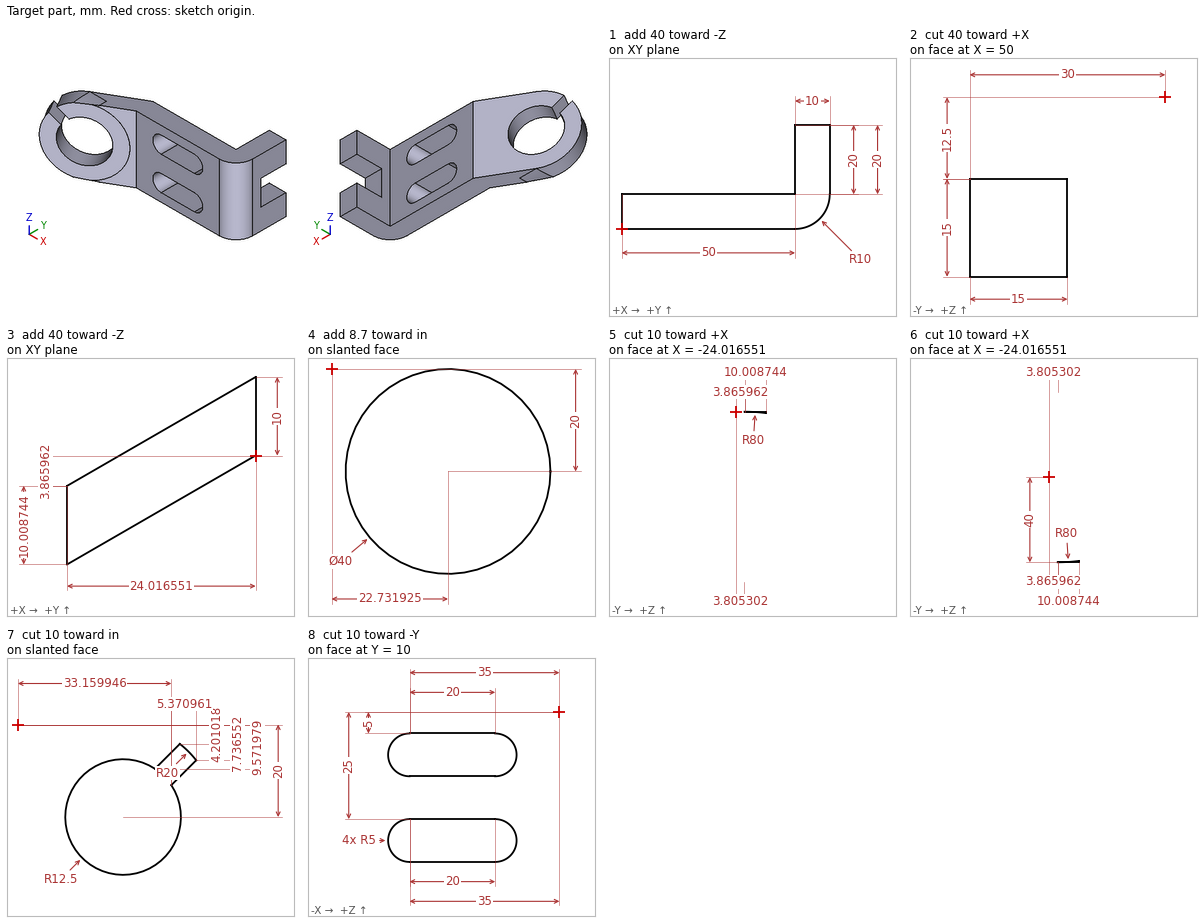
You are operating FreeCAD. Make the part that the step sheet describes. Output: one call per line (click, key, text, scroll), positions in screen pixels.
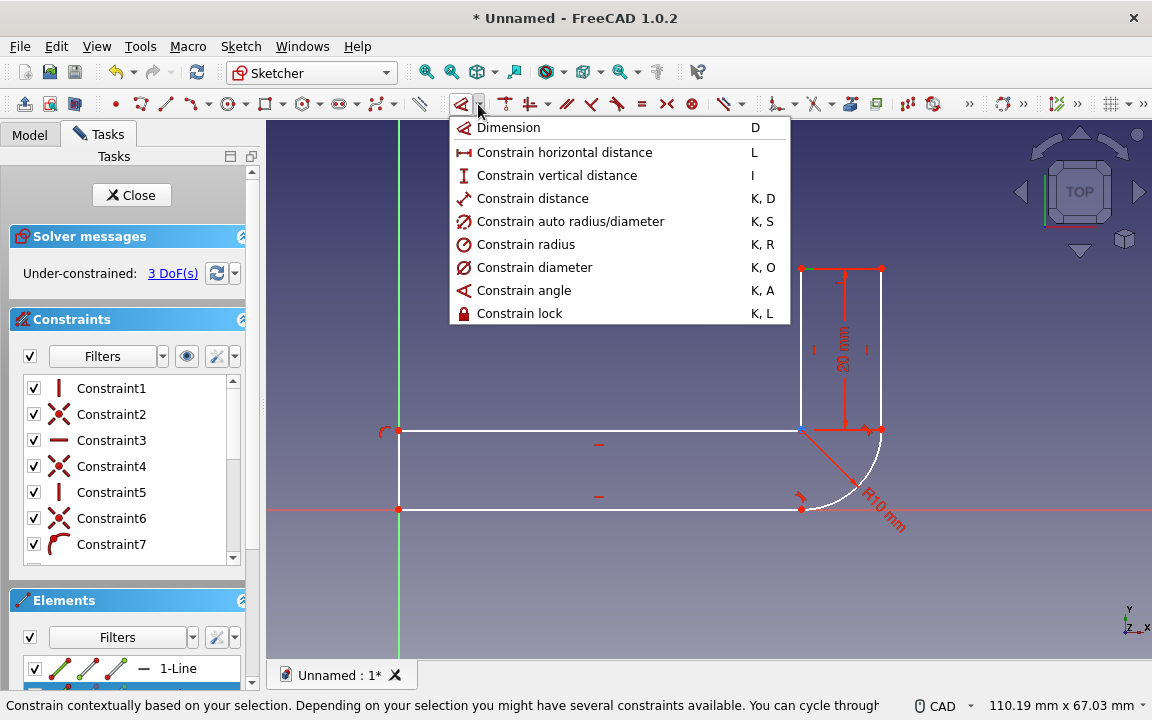
click(620, 152)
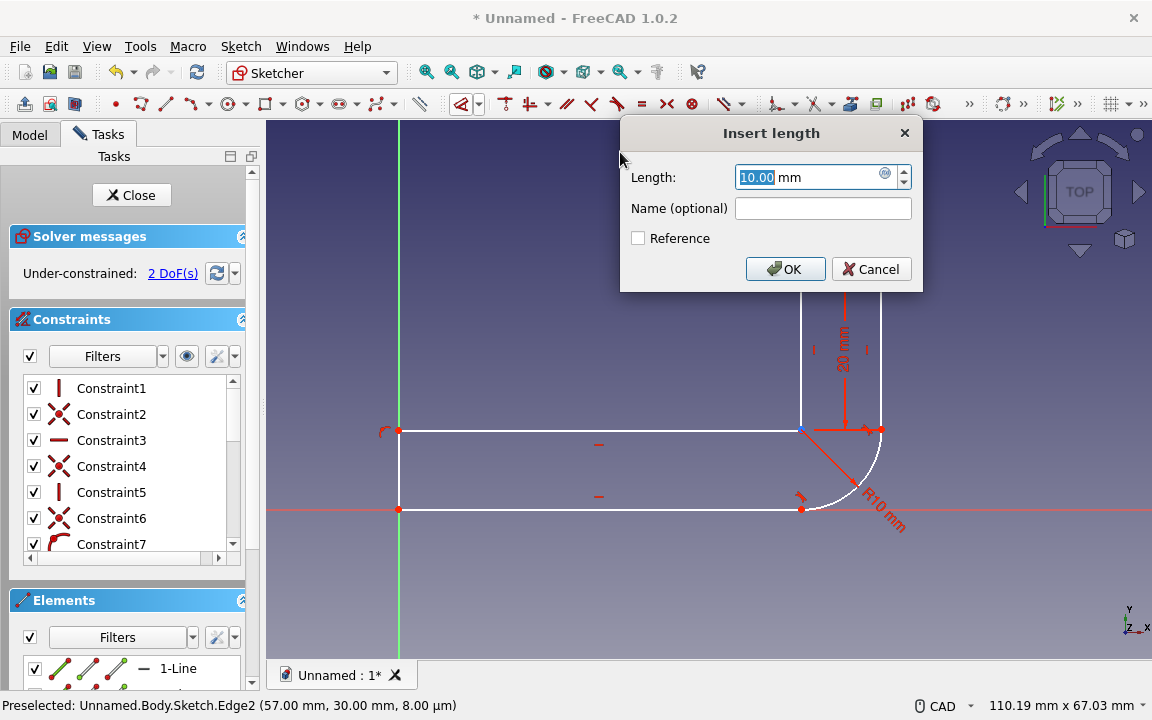
text(10)
key(Return)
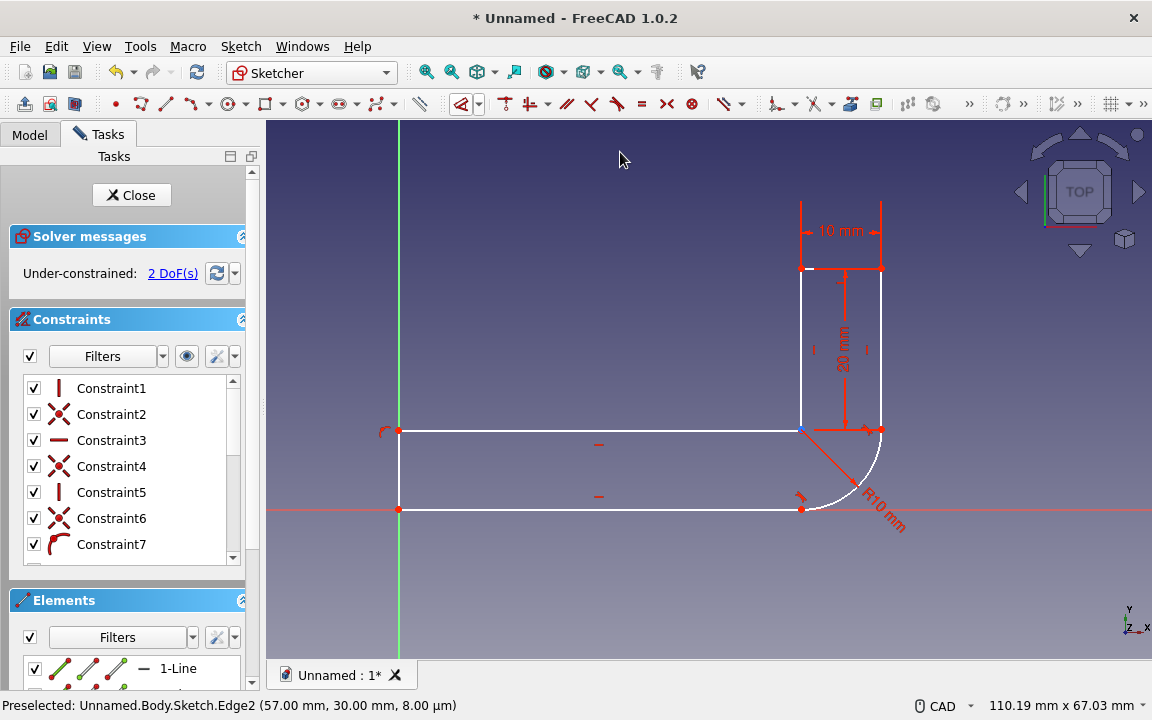
click(801, 317)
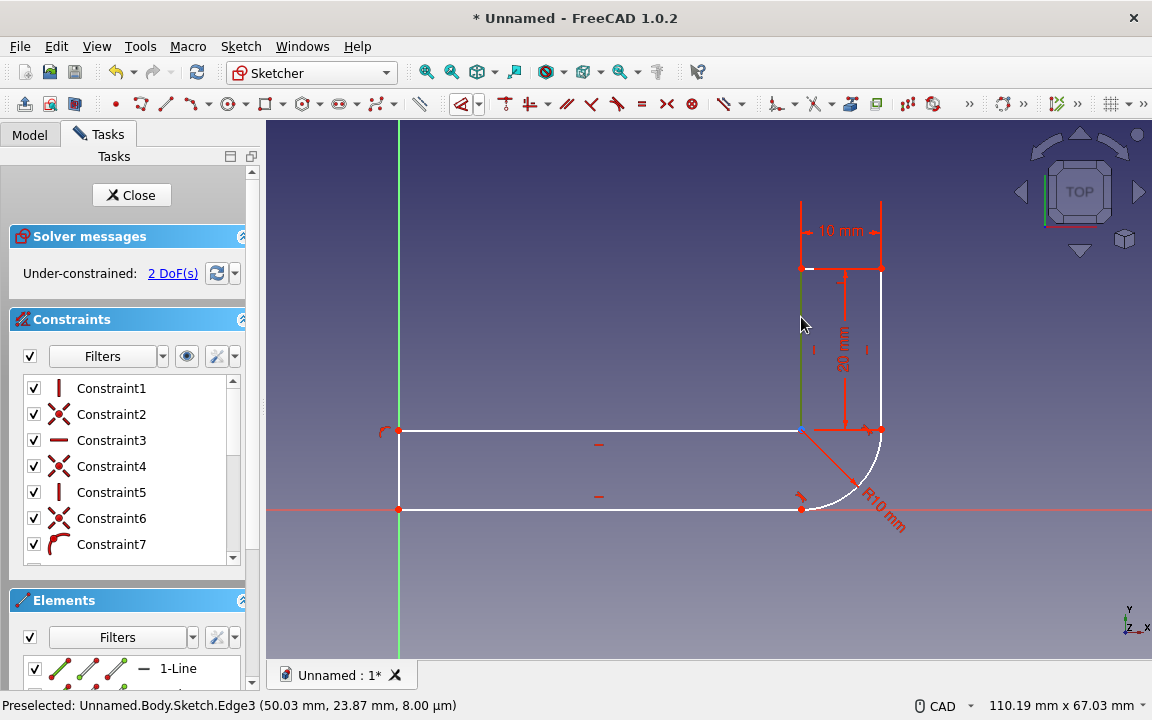
click(478, 104)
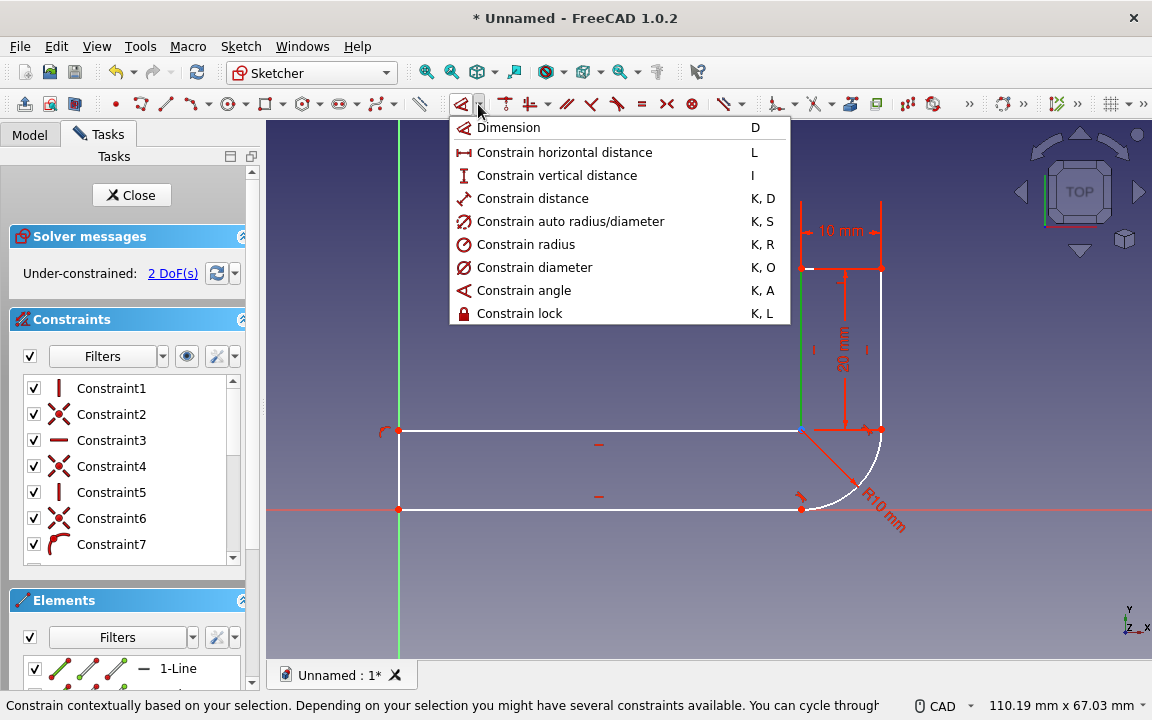
click(620, 176)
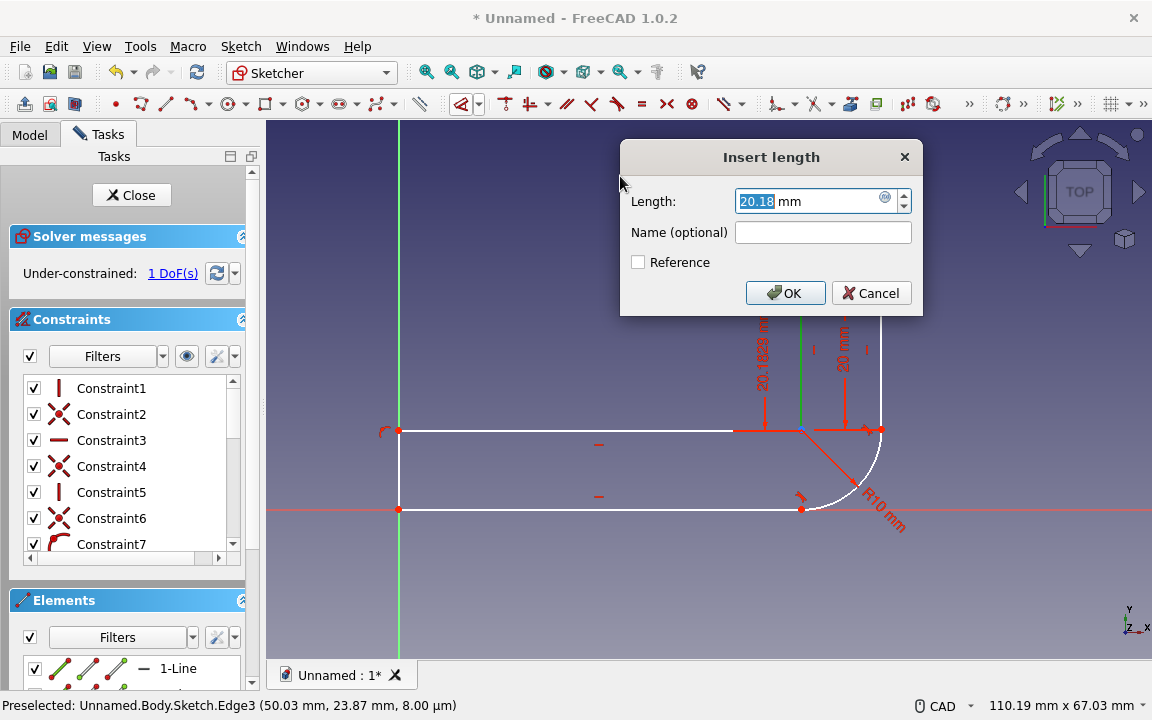
text(20)
key(Return)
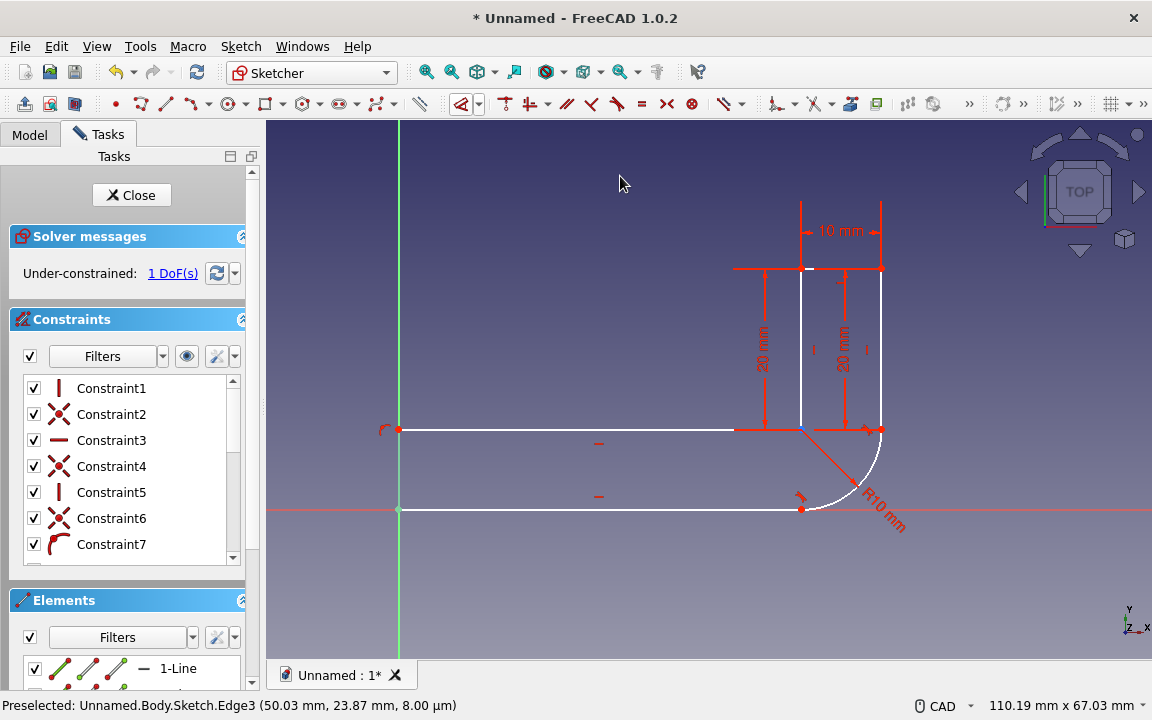
click(680, 430)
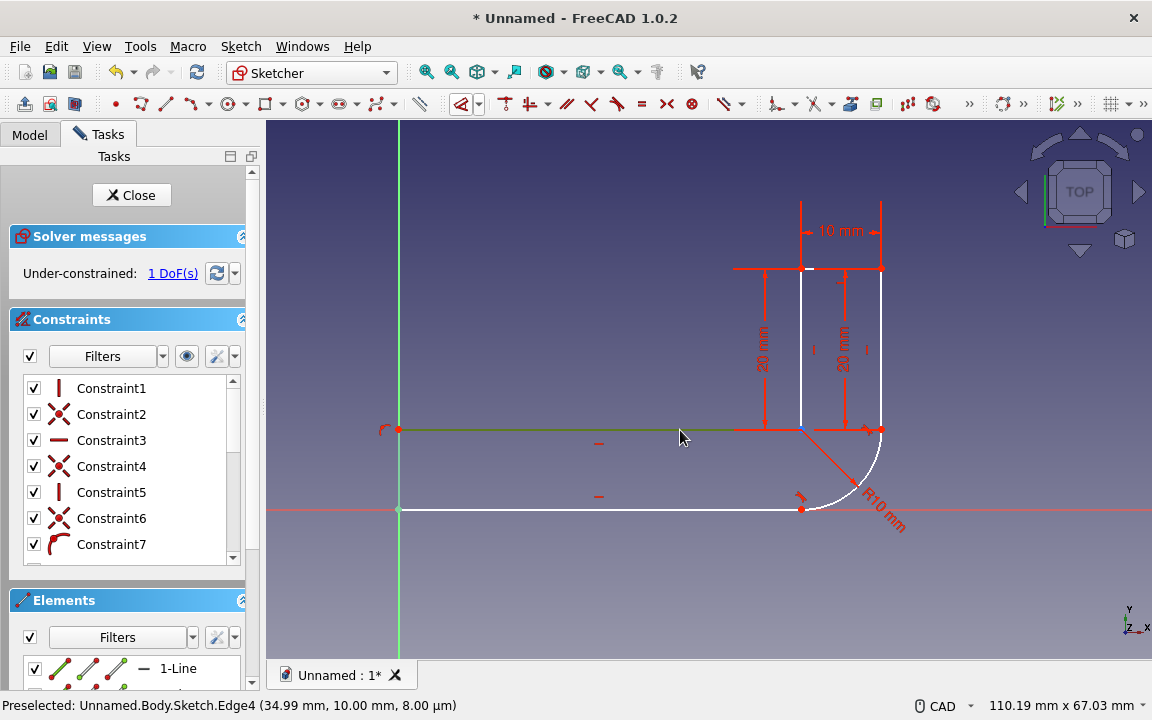
click(478, 104)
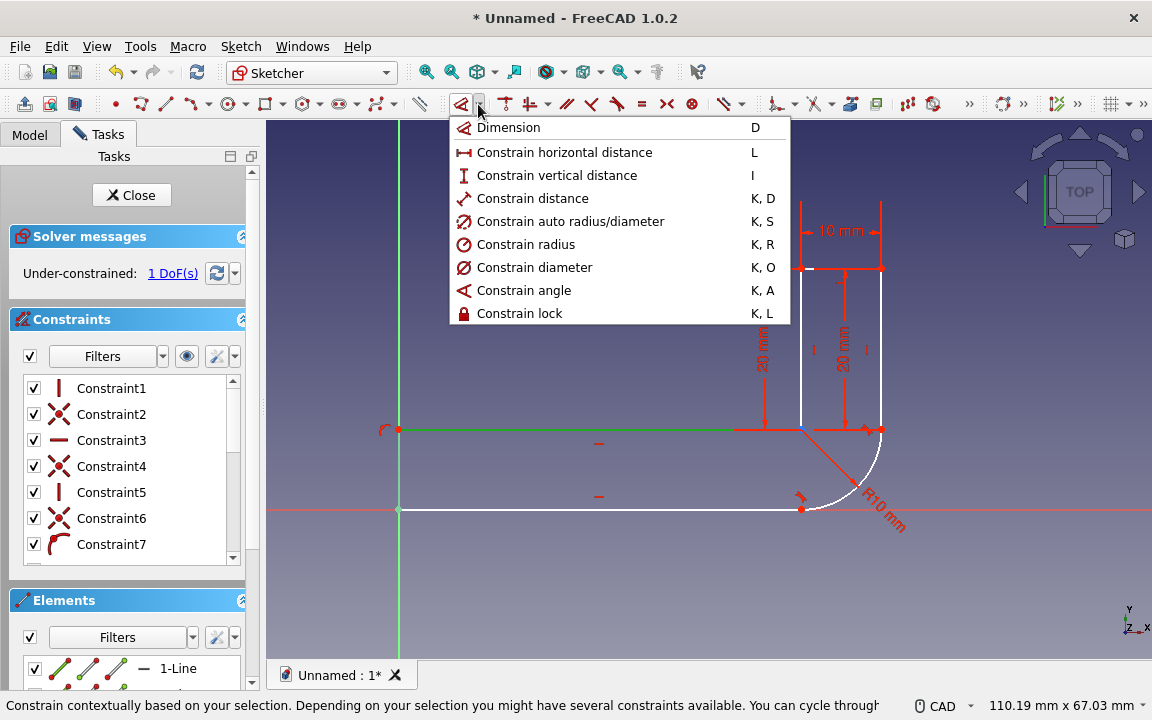
click(620, 152)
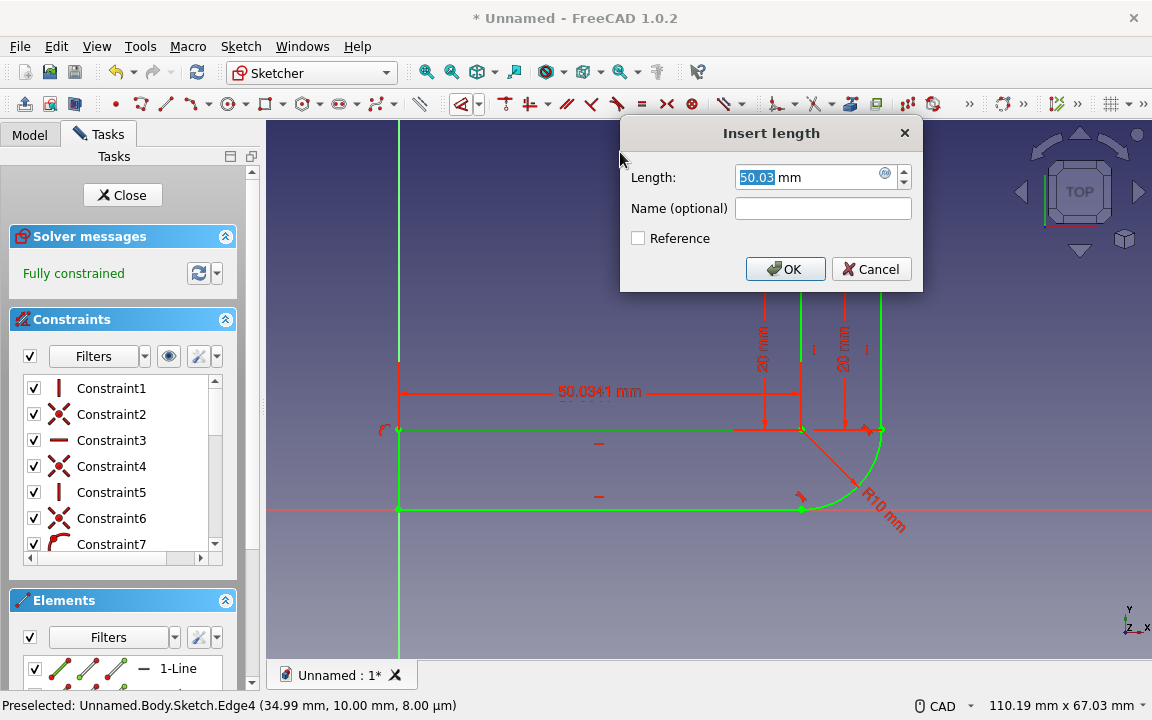
text(50)
key(Return)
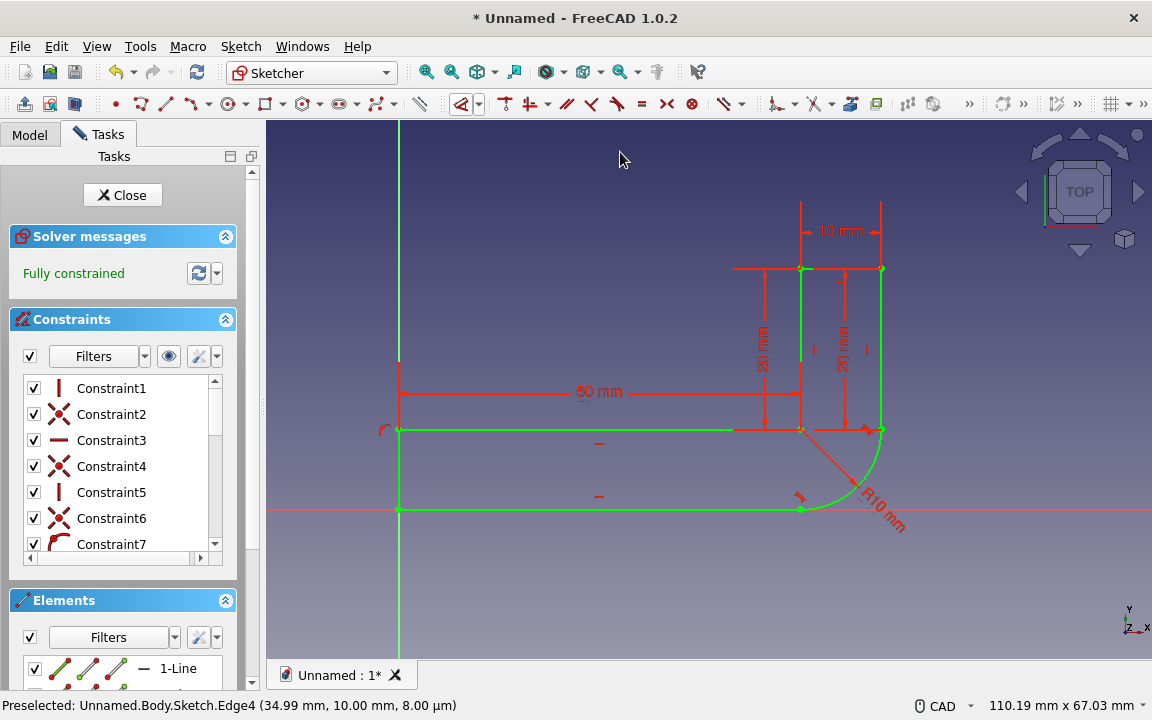
click(123, 195)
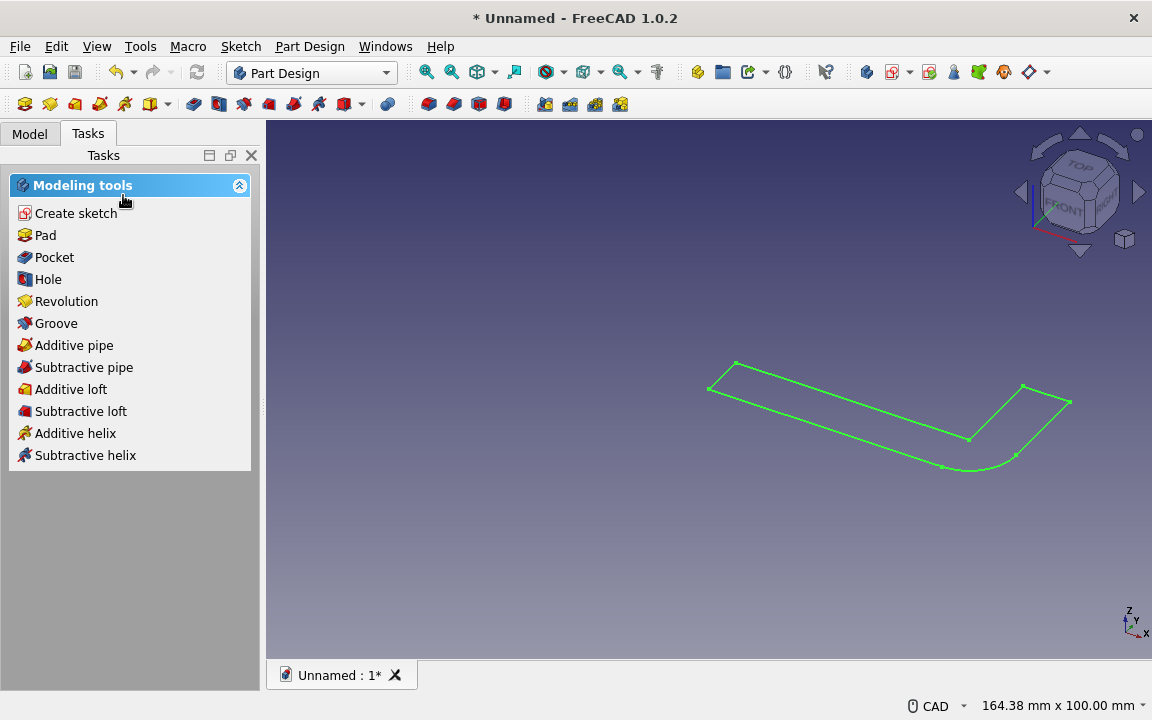
click(25, 104)